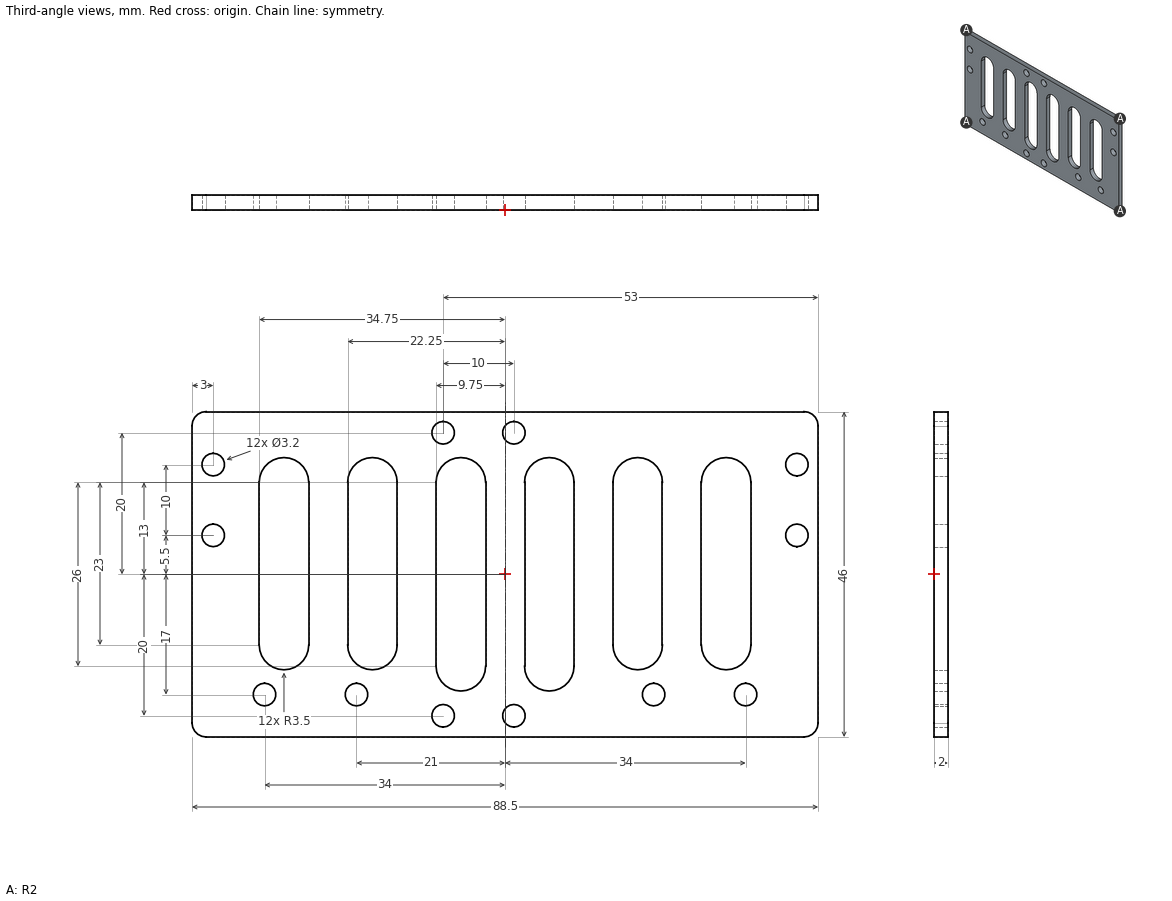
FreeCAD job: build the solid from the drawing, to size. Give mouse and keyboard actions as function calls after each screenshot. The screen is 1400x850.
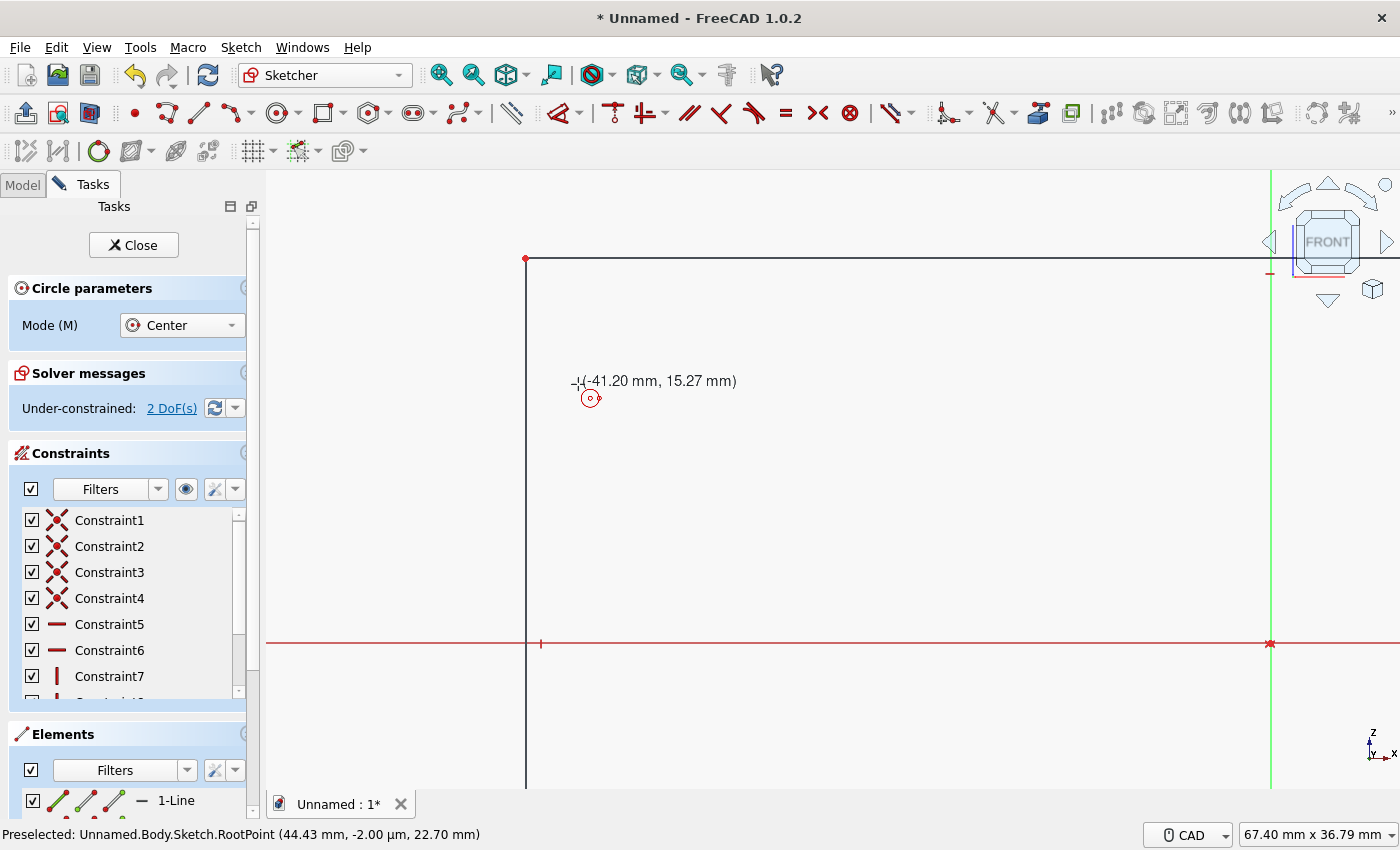
click(577, 382)
click(596, 363)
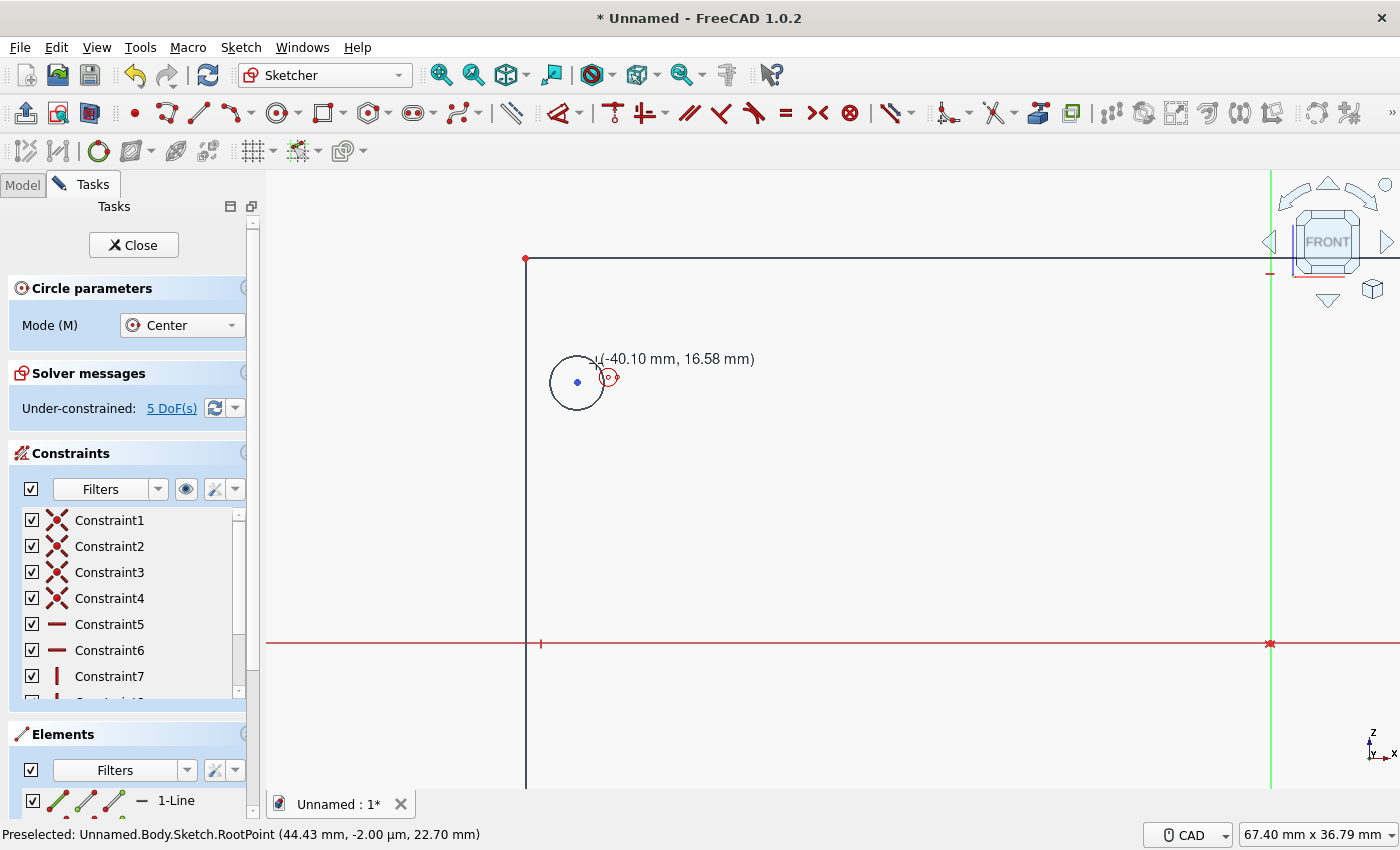
click(1123, 306)
click(1142, 287)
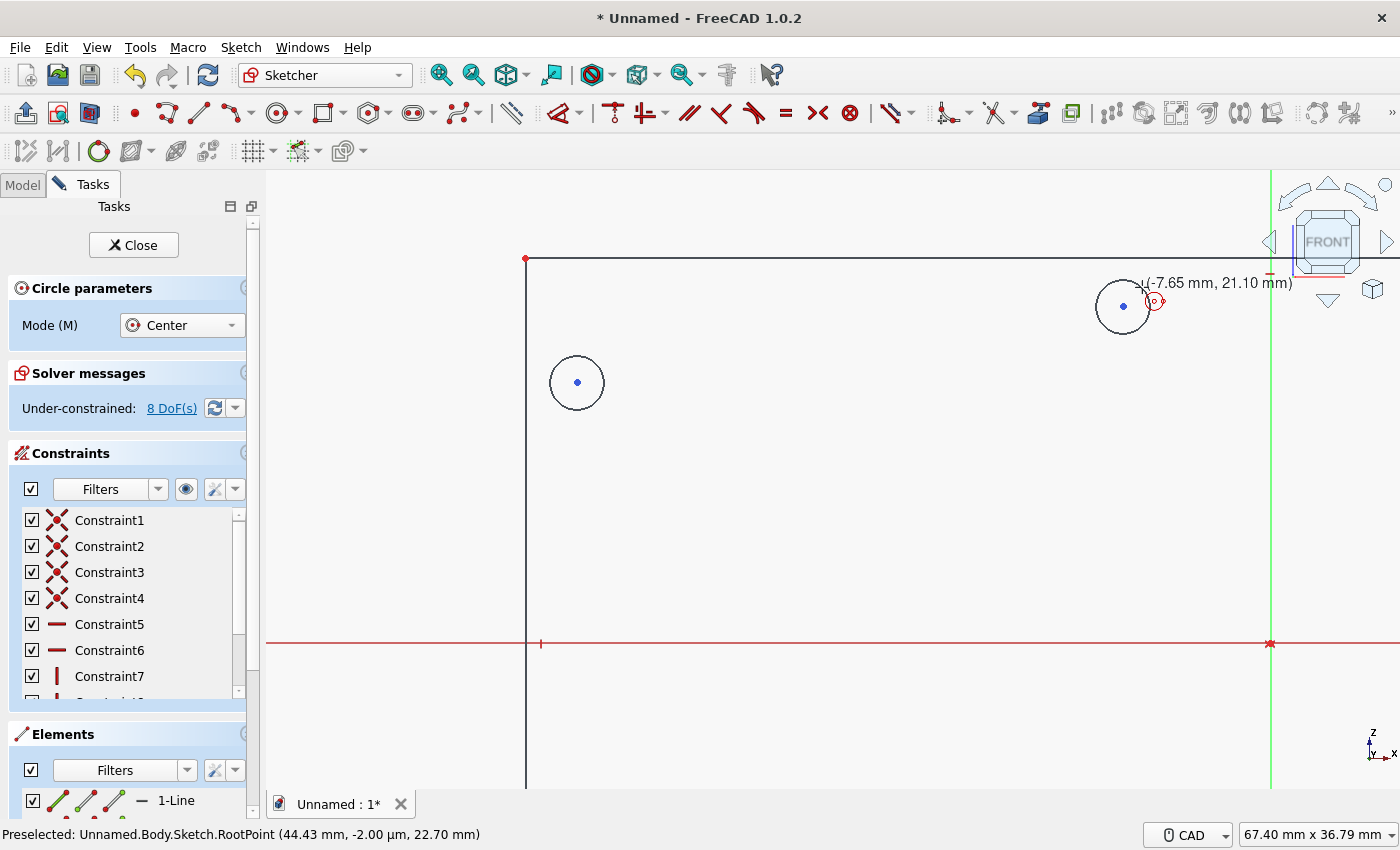
click(577, 550)
click(596, 531)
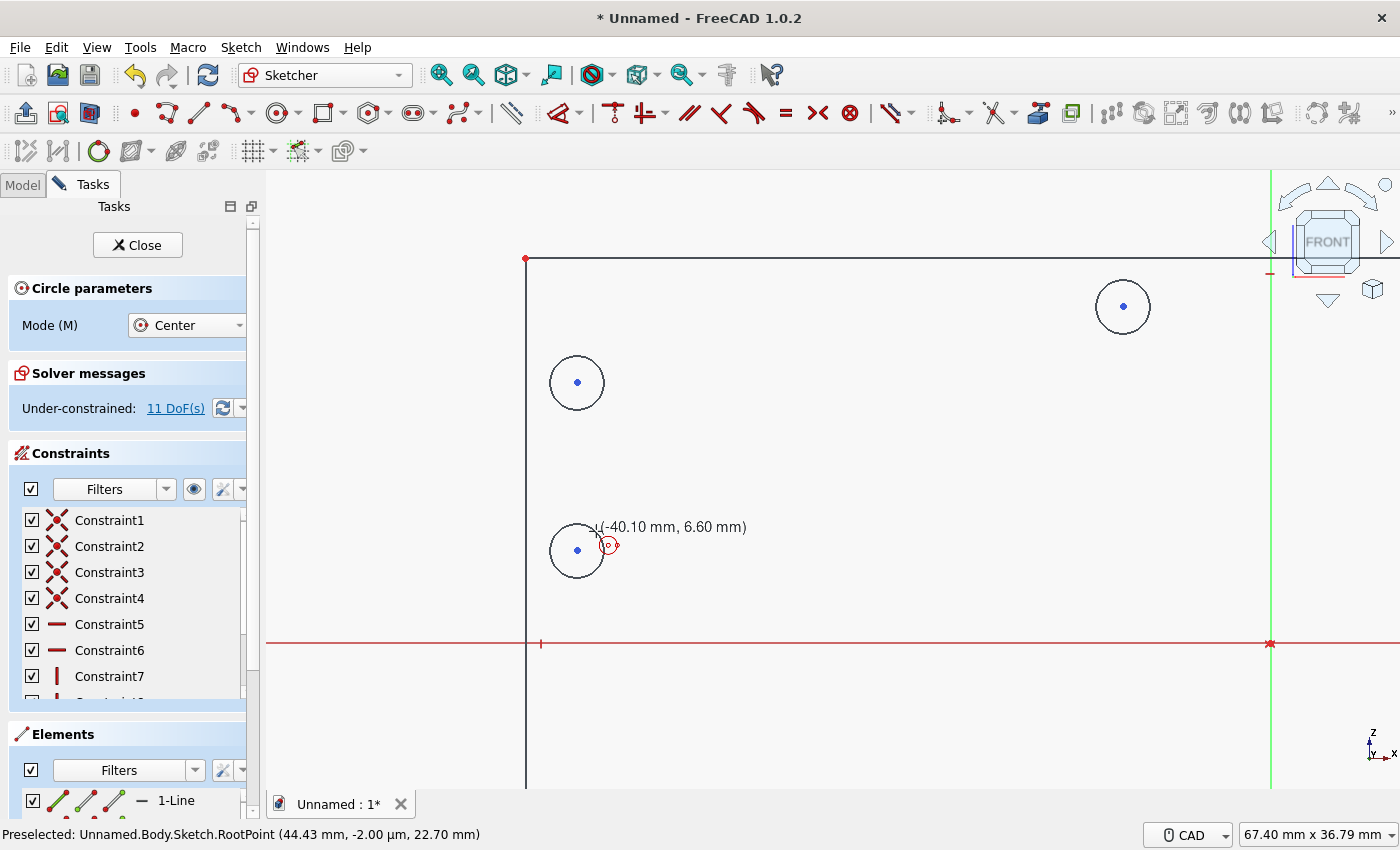
scroll(351, 346, down, 4)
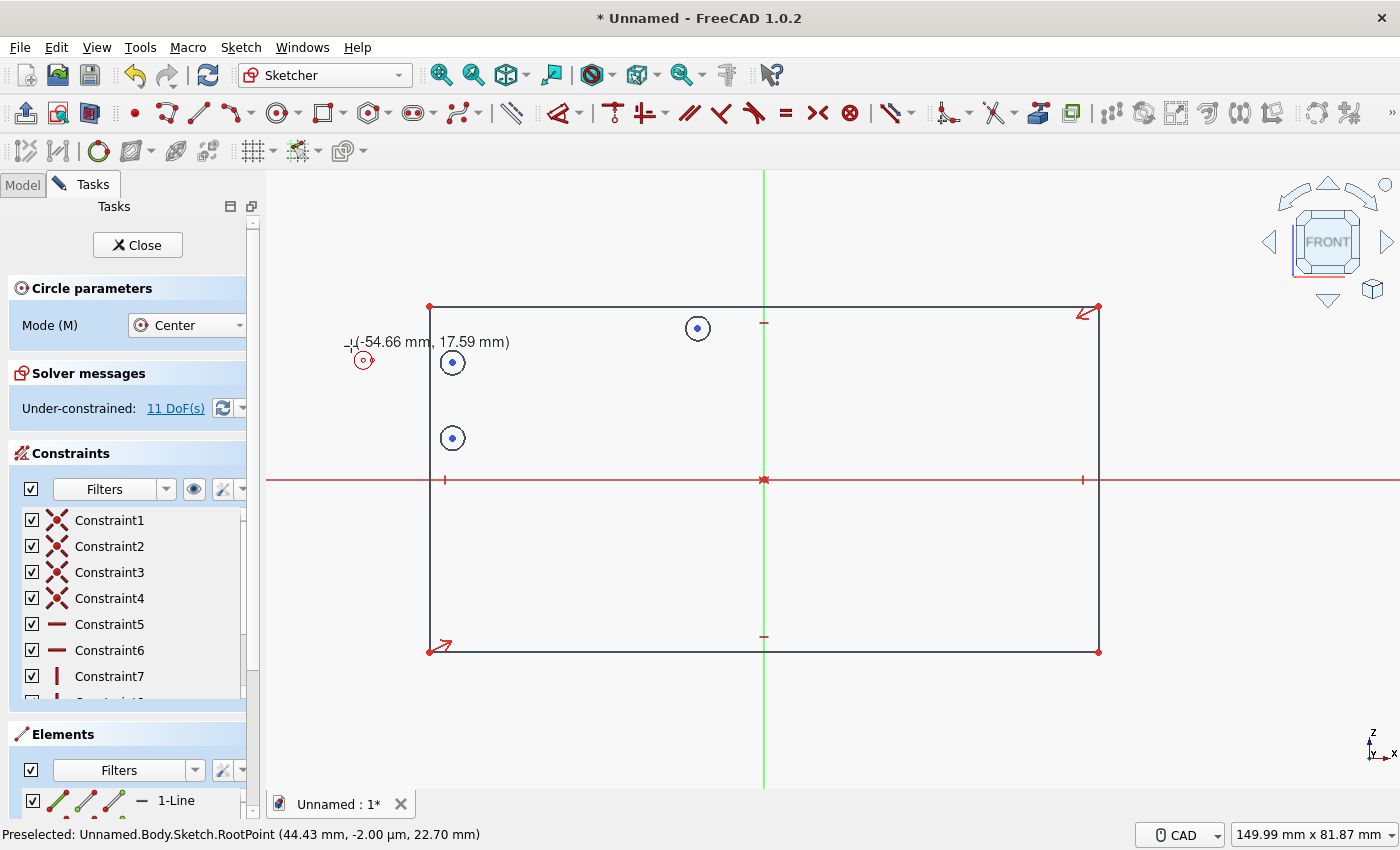
scroll(774, 328, up, 4)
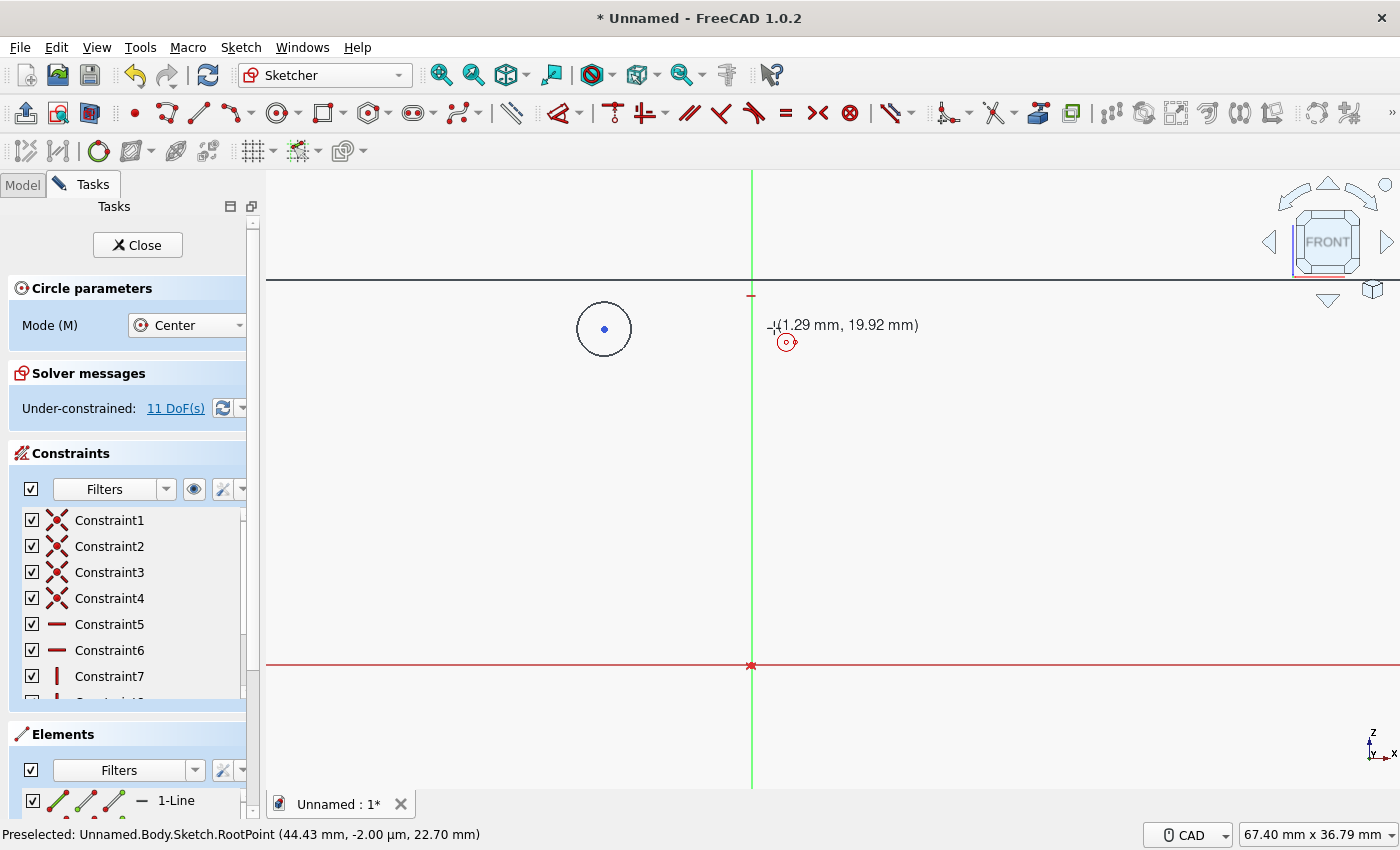
click(773, 329)
click(792, 310)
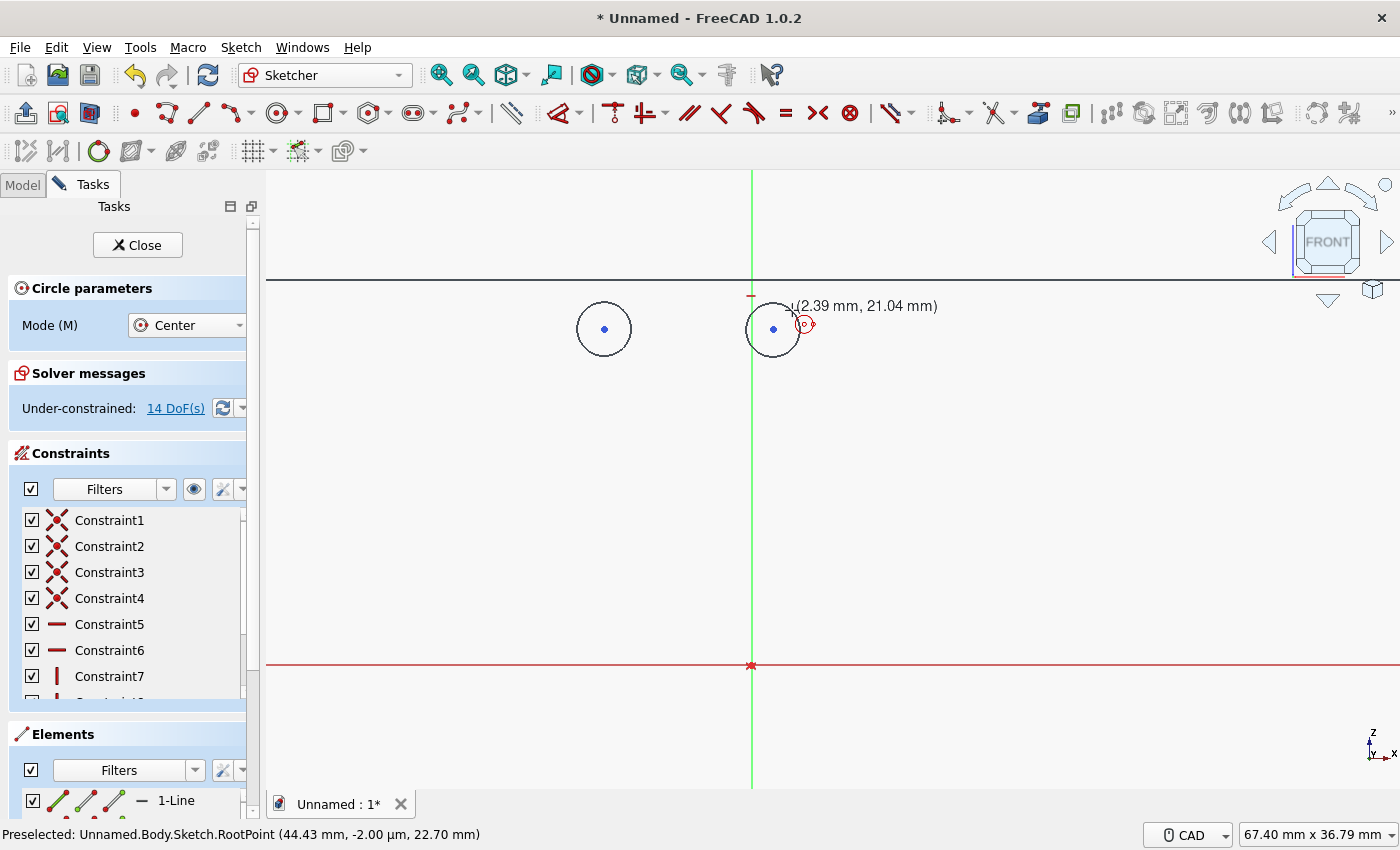
scroll(775, 328, down, 4)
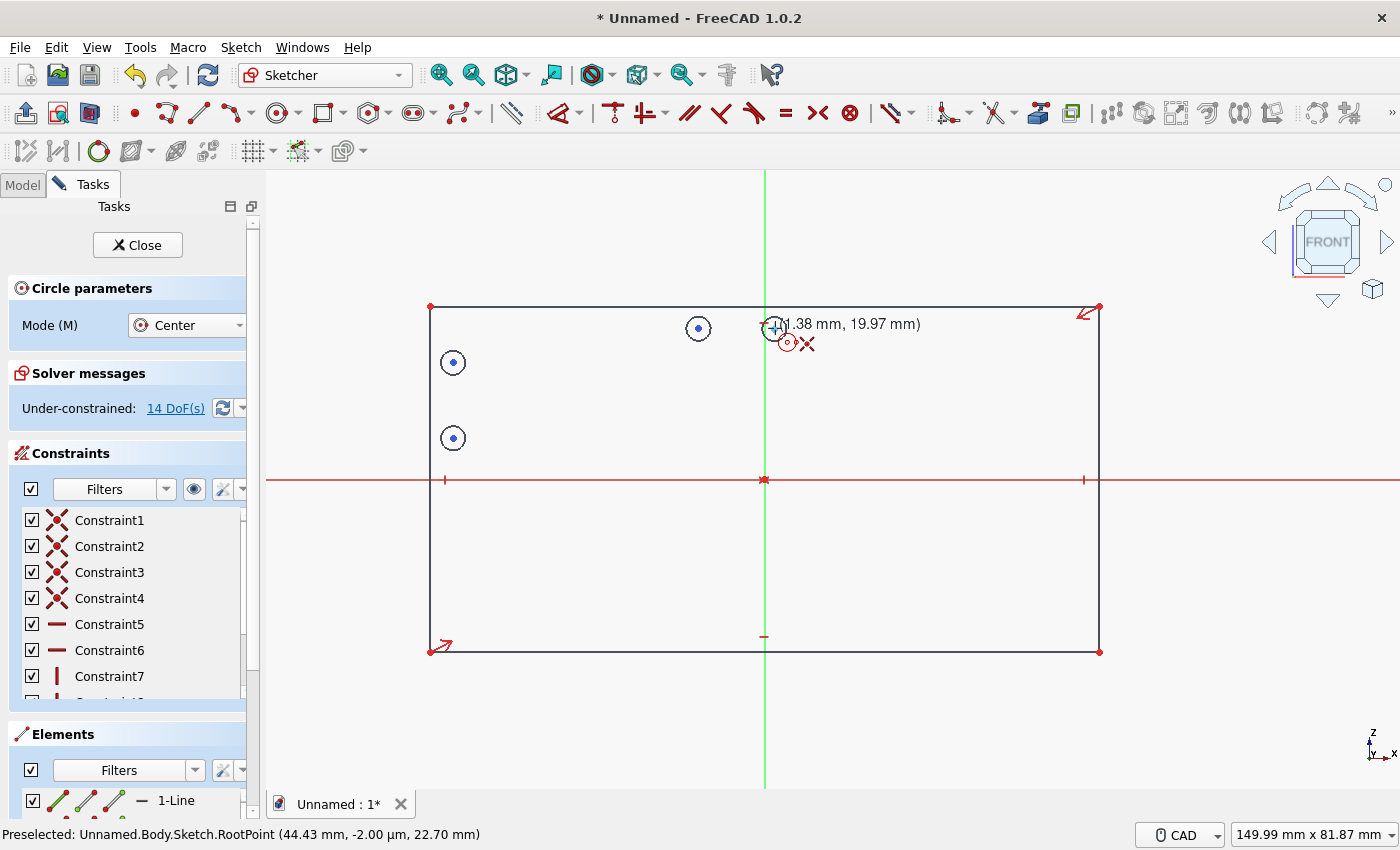
scroll(1077, 362, up, 4)